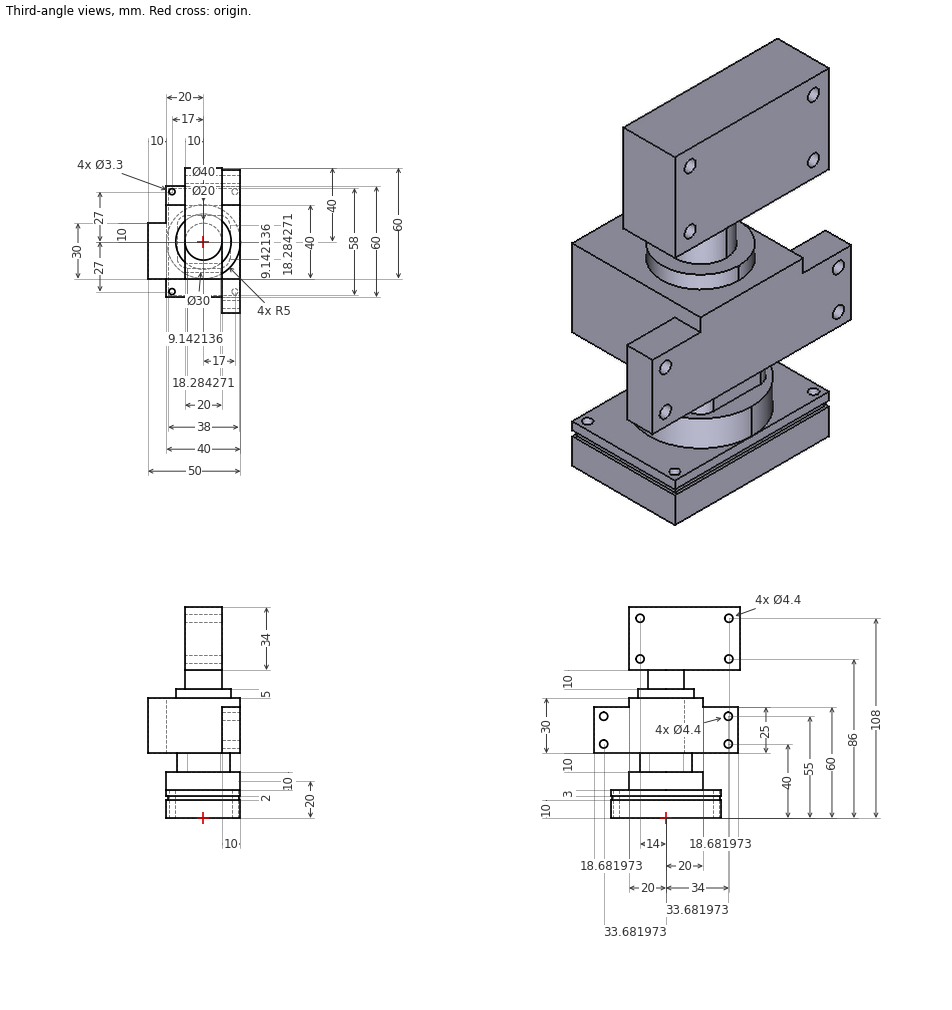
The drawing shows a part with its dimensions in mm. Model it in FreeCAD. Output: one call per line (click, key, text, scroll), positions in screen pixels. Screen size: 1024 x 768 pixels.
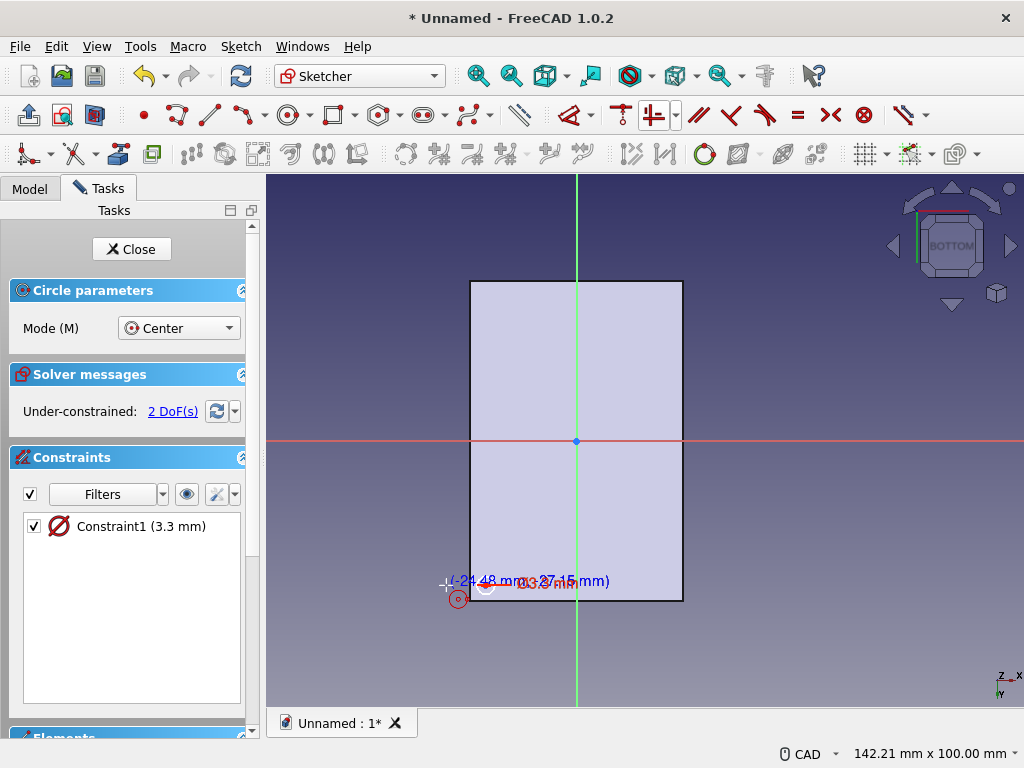
scroll(486, 297, up, 5)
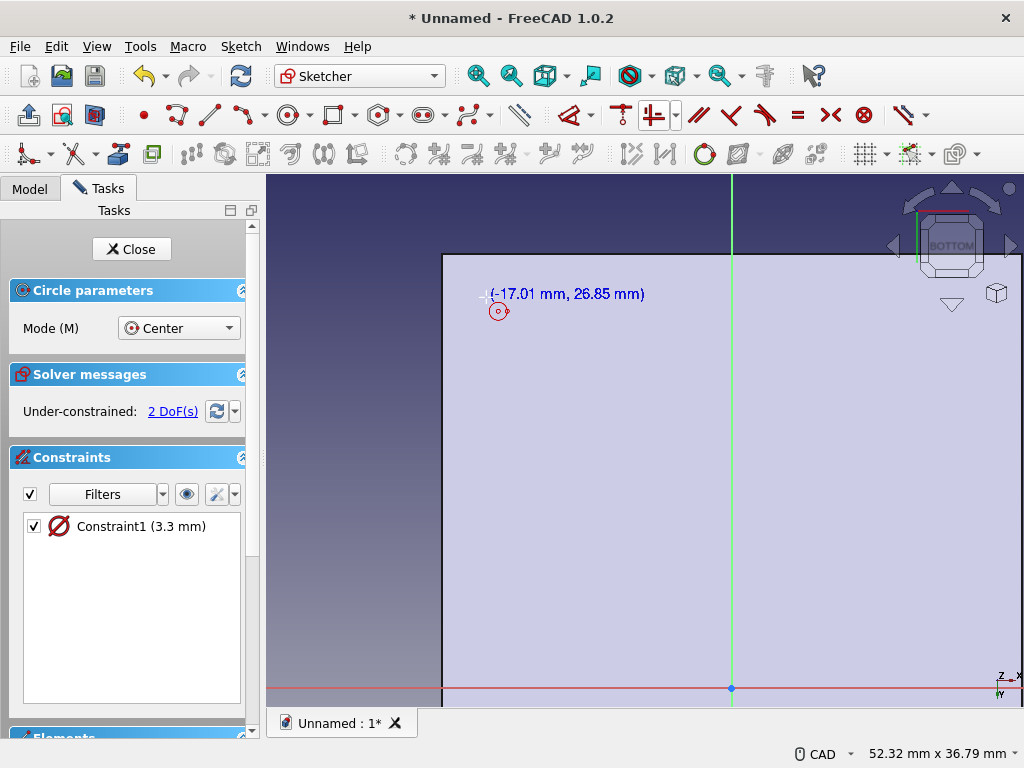
click(486, 297)
move(502, 280)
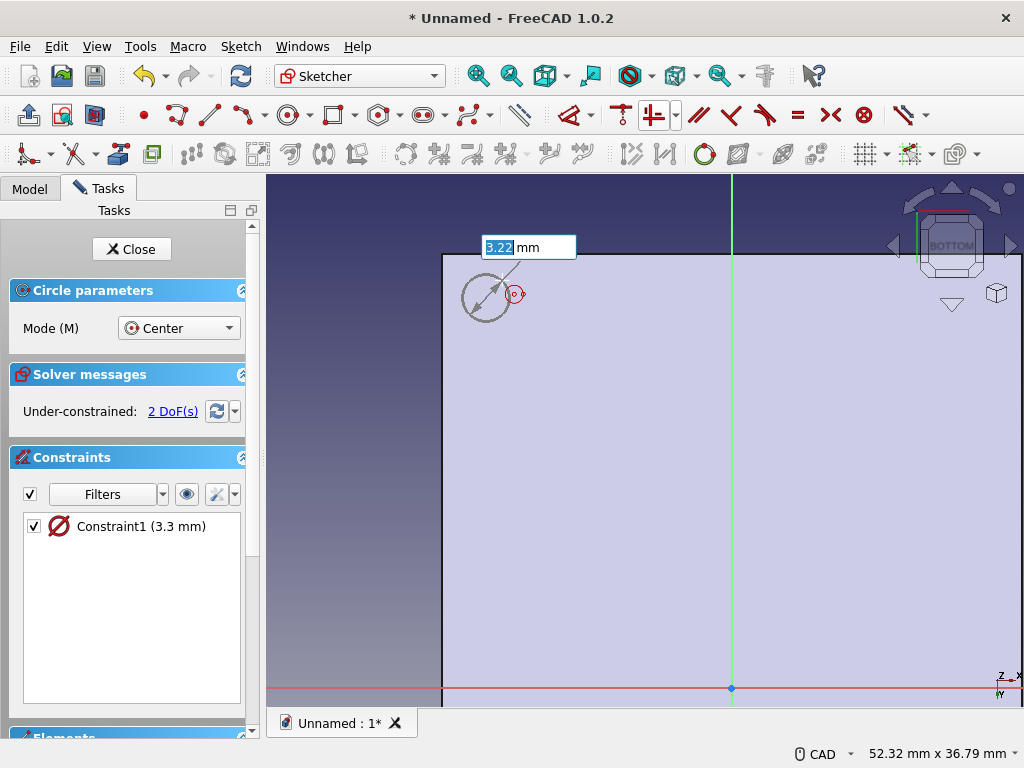
text(3.3)
key(Return)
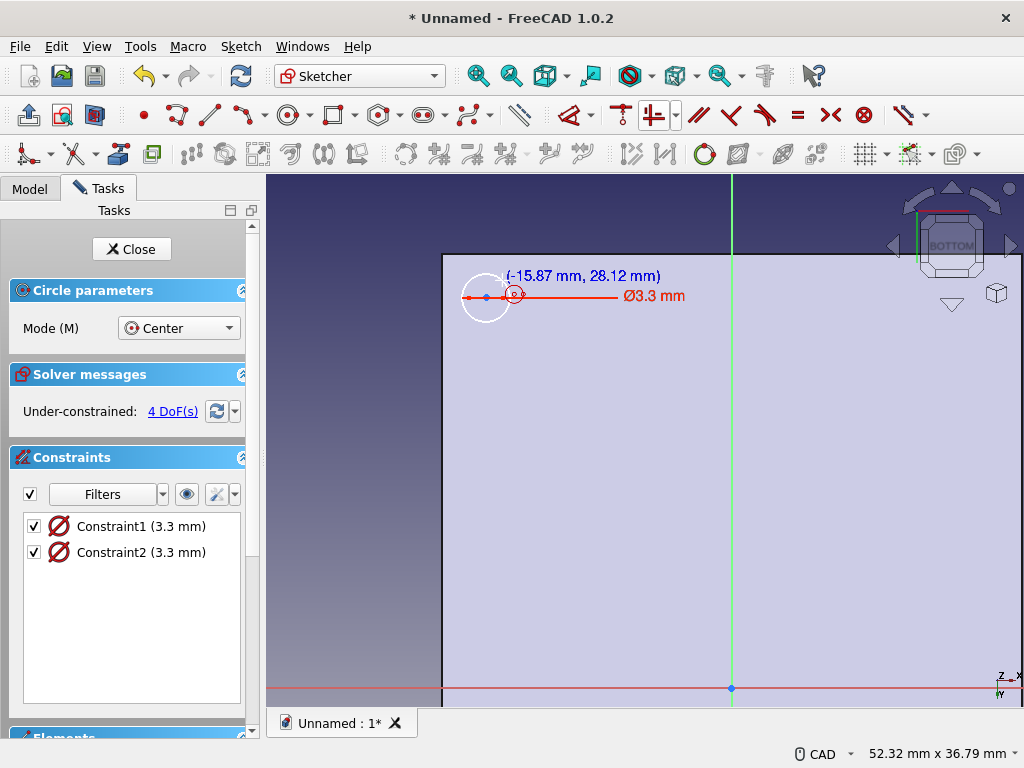
scroll(486, 296, down, 5)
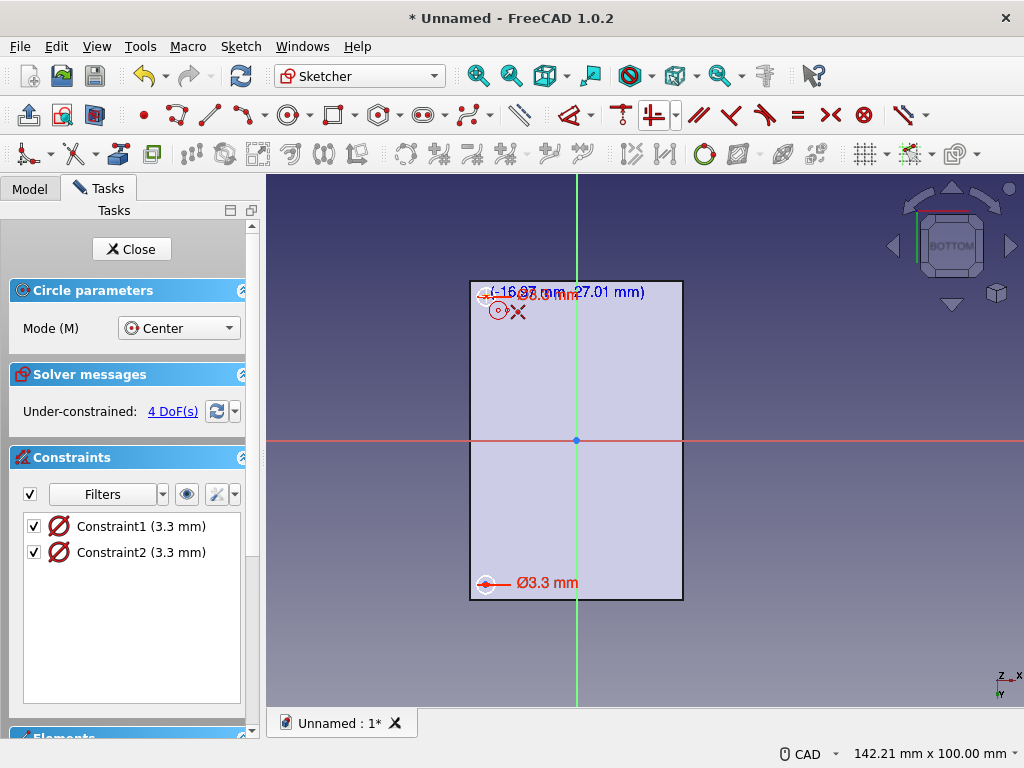
scroll(667, 297, up, 5)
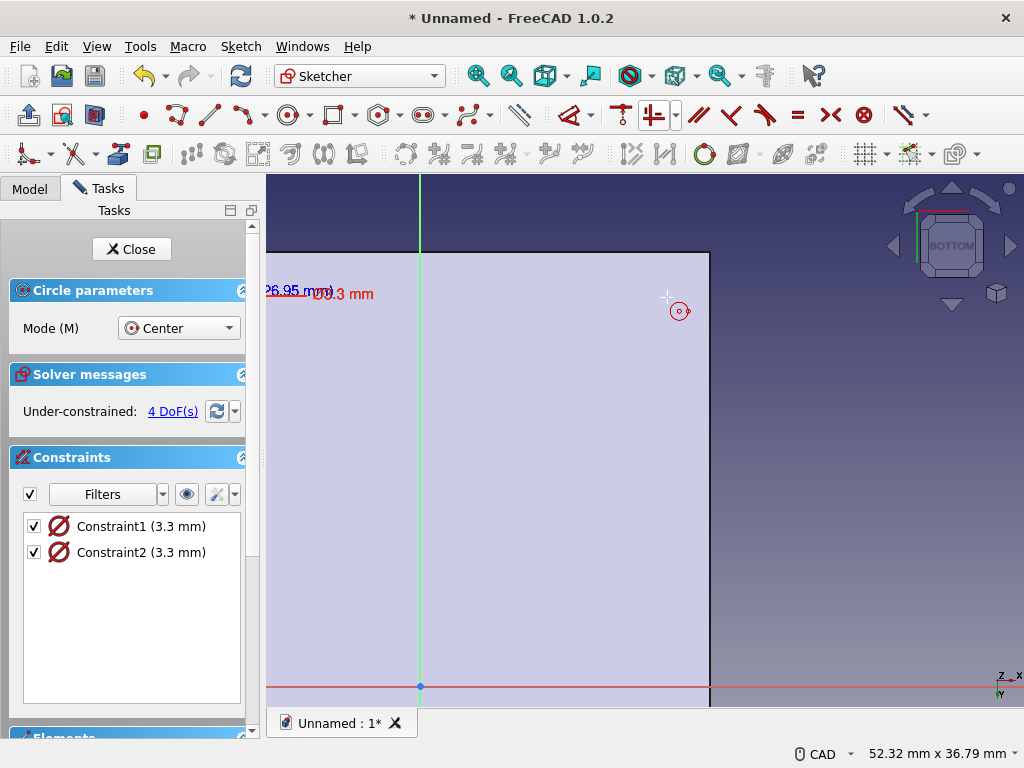
click(667, 295)
move(684, 279)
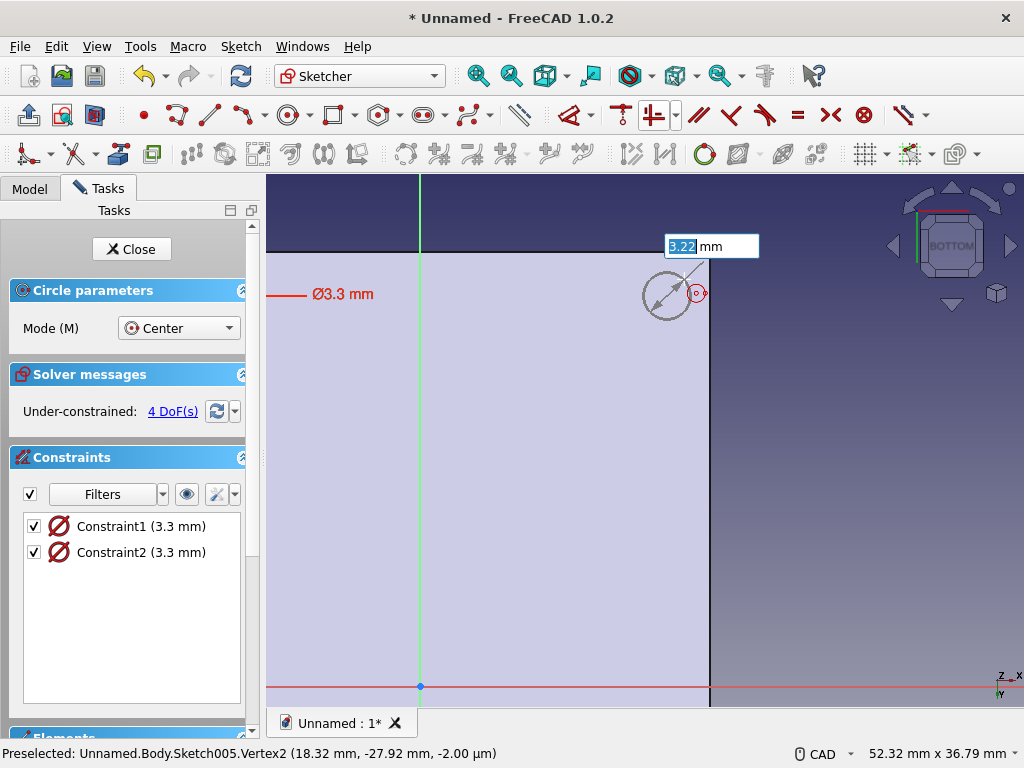
text(3.3)
key(Return)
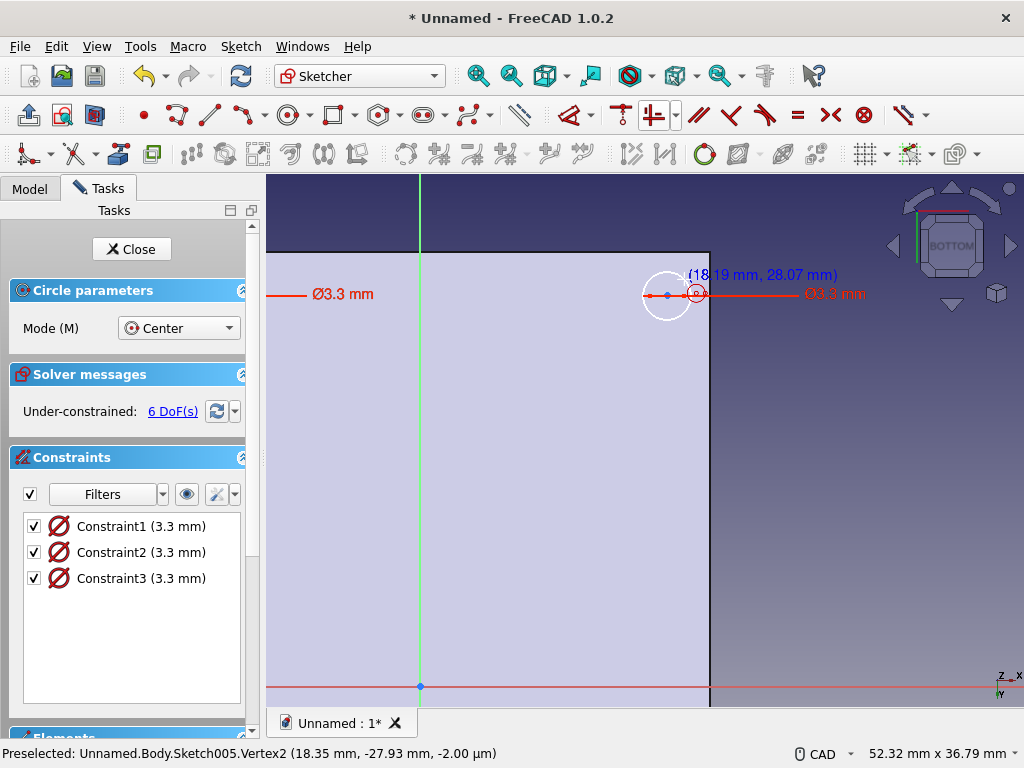
scroll(667, 297, down, 5)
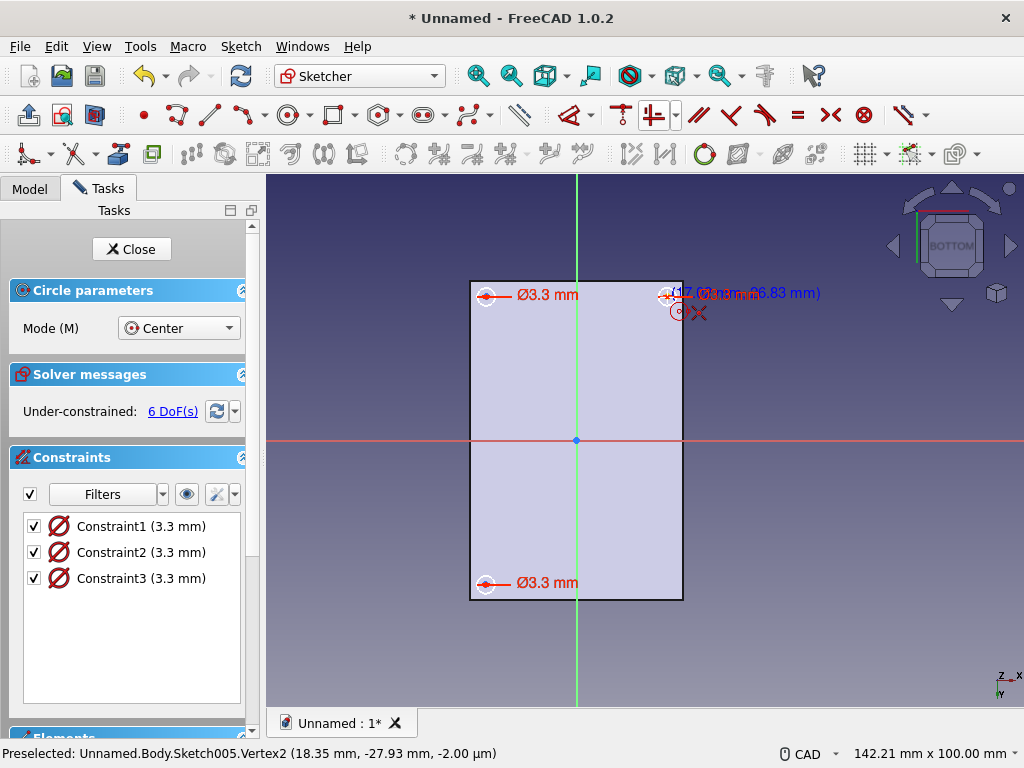
scroll(667, 584, up, 5)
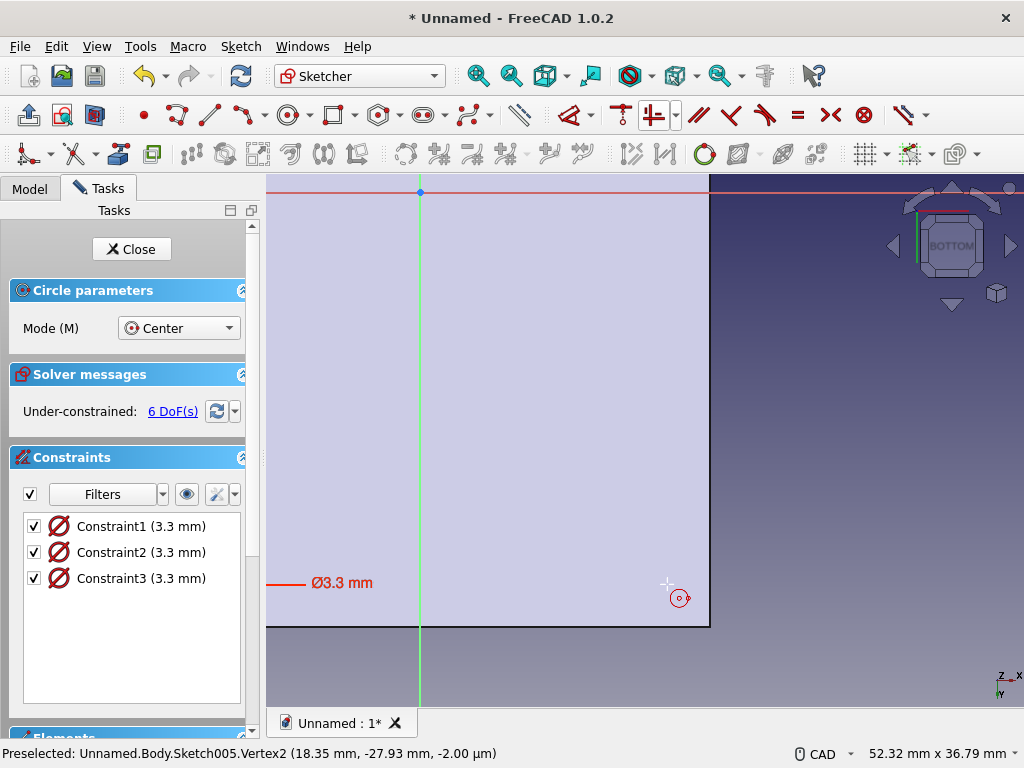
click(667, 584)
move(684, 567)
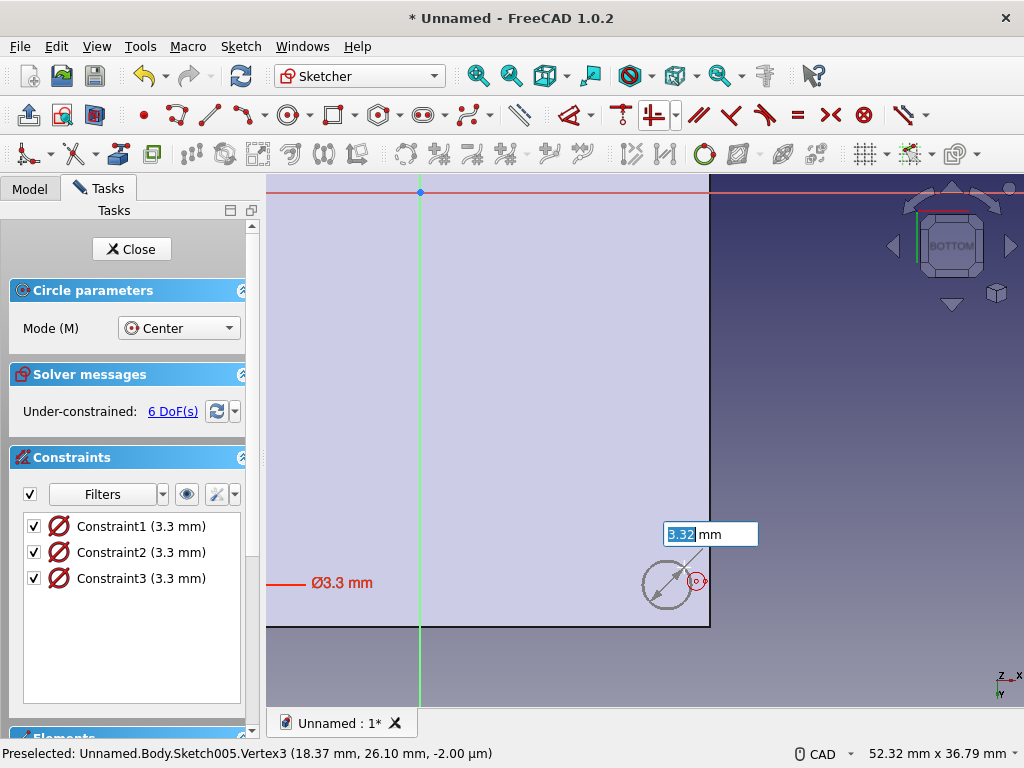
text(3.3)
key(Return)
key(Escape)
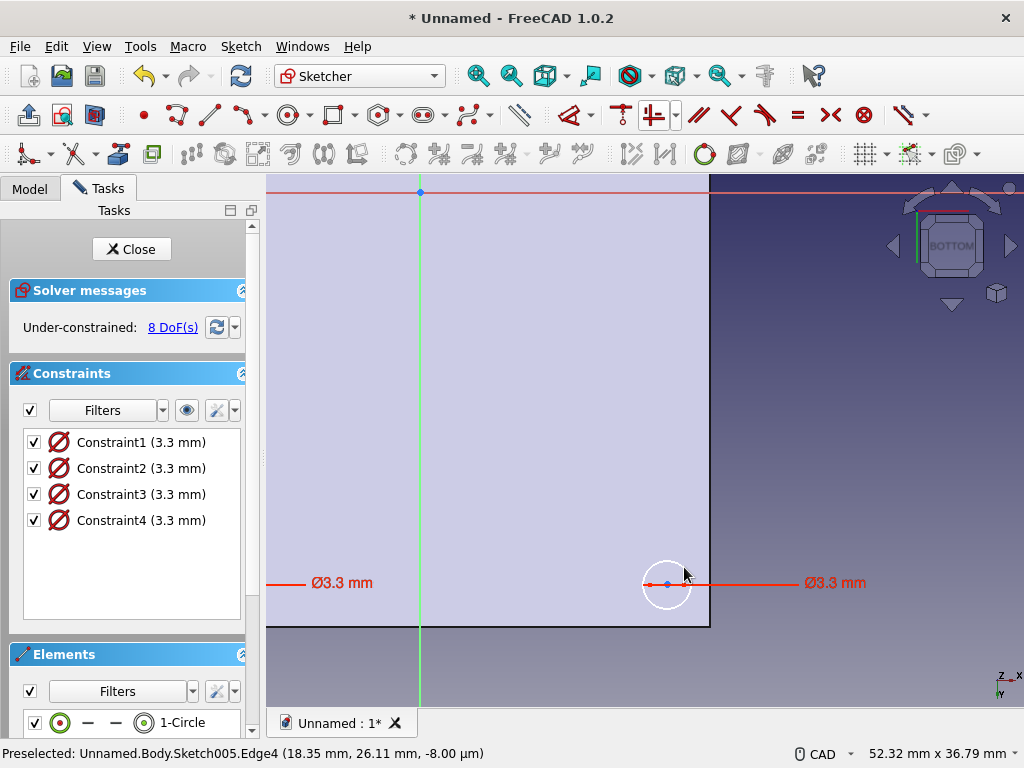
scroll(667, 585, down, 5)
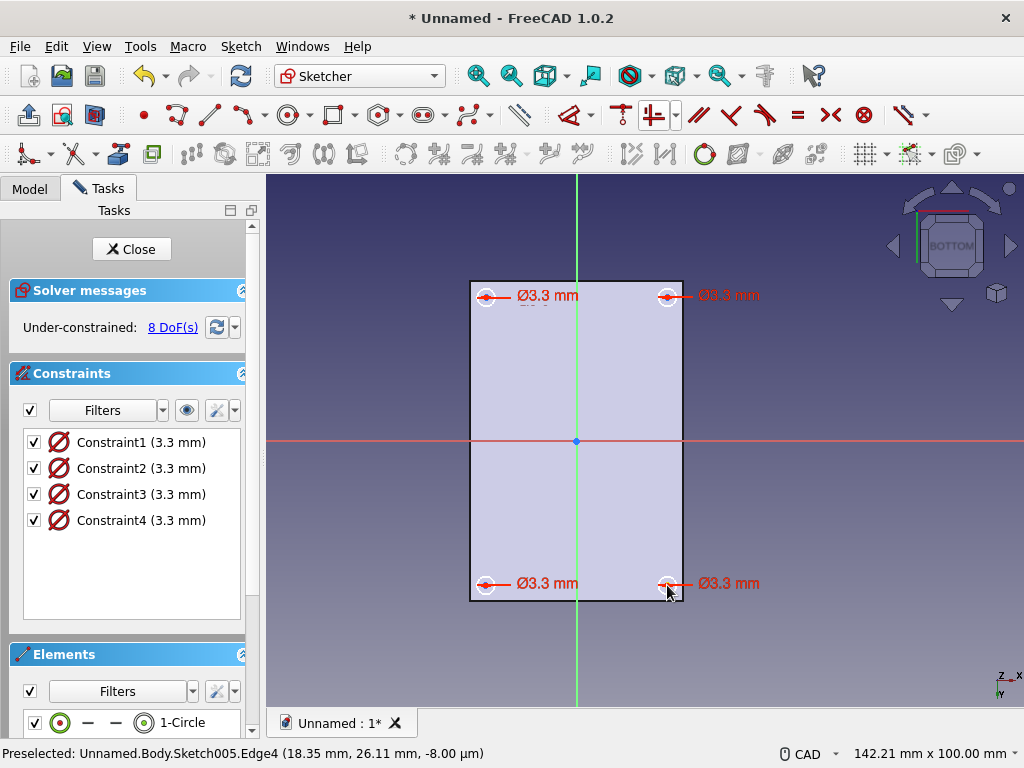
click(486, 585)